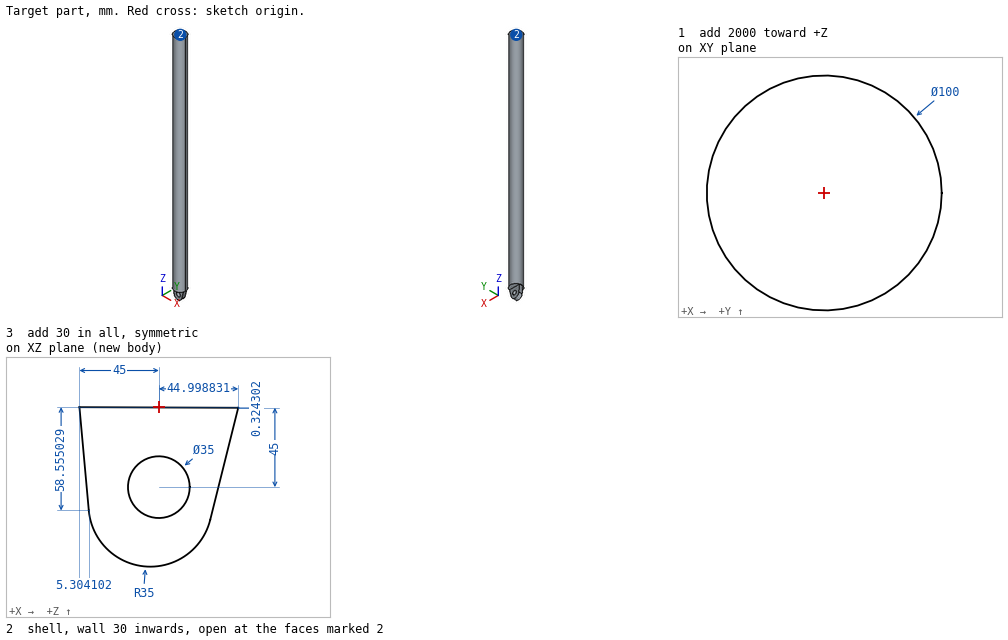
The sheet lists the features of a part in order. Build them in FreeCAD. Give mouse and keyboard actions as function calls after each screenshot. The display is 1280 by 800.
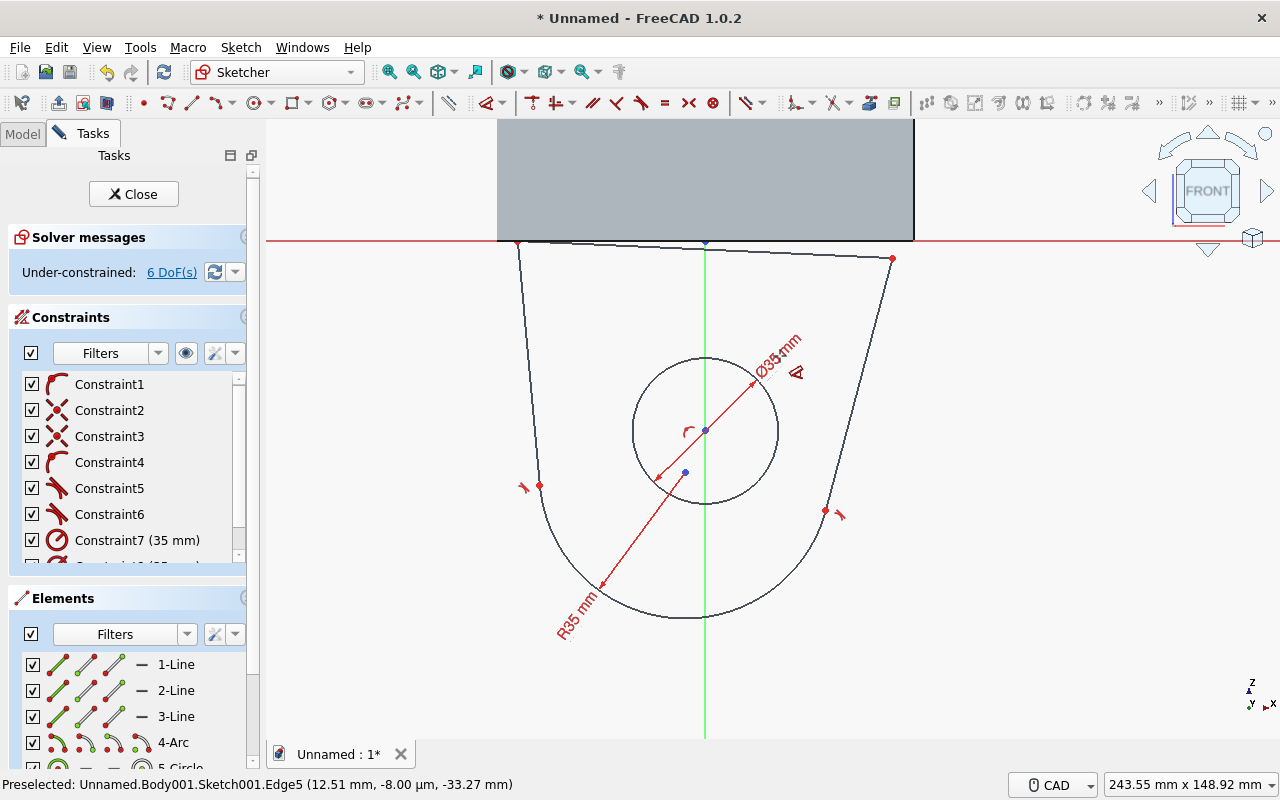
click(518, 241)
click(612, 207)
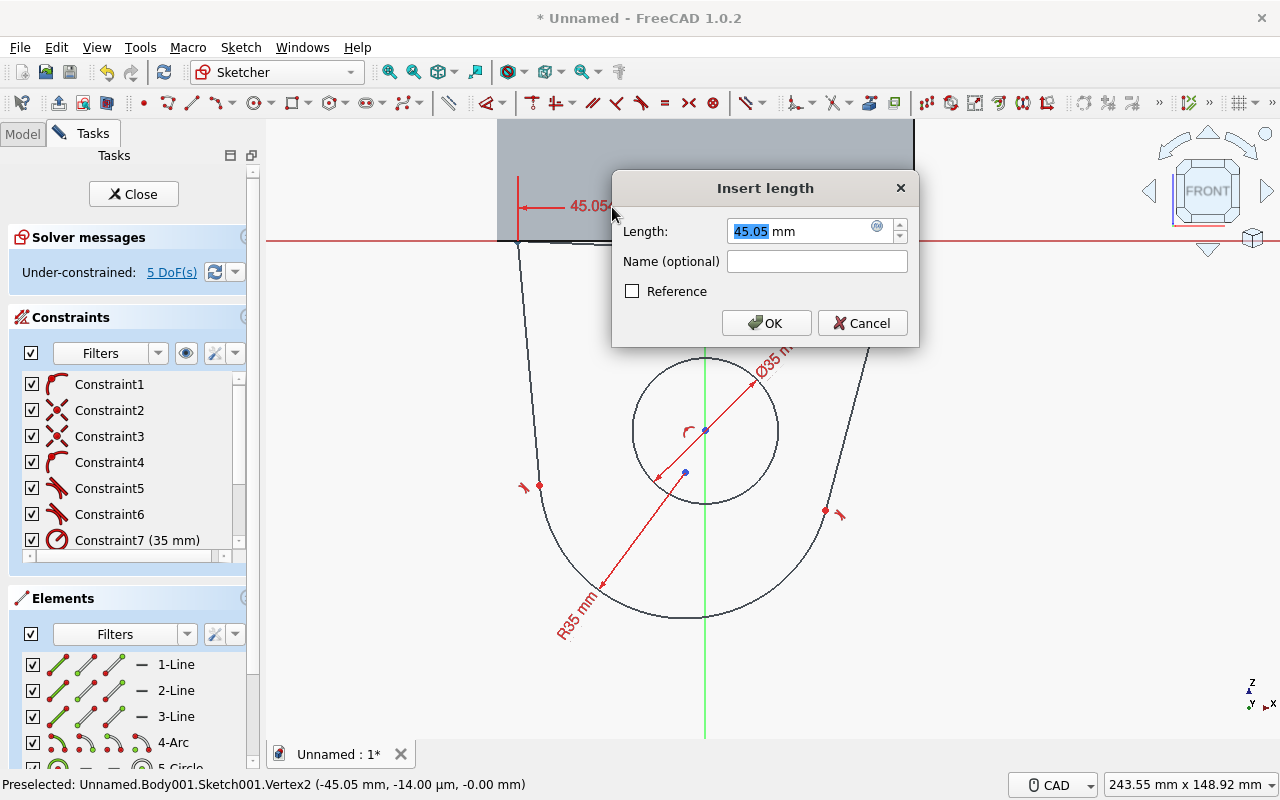
text(45)
key(Return)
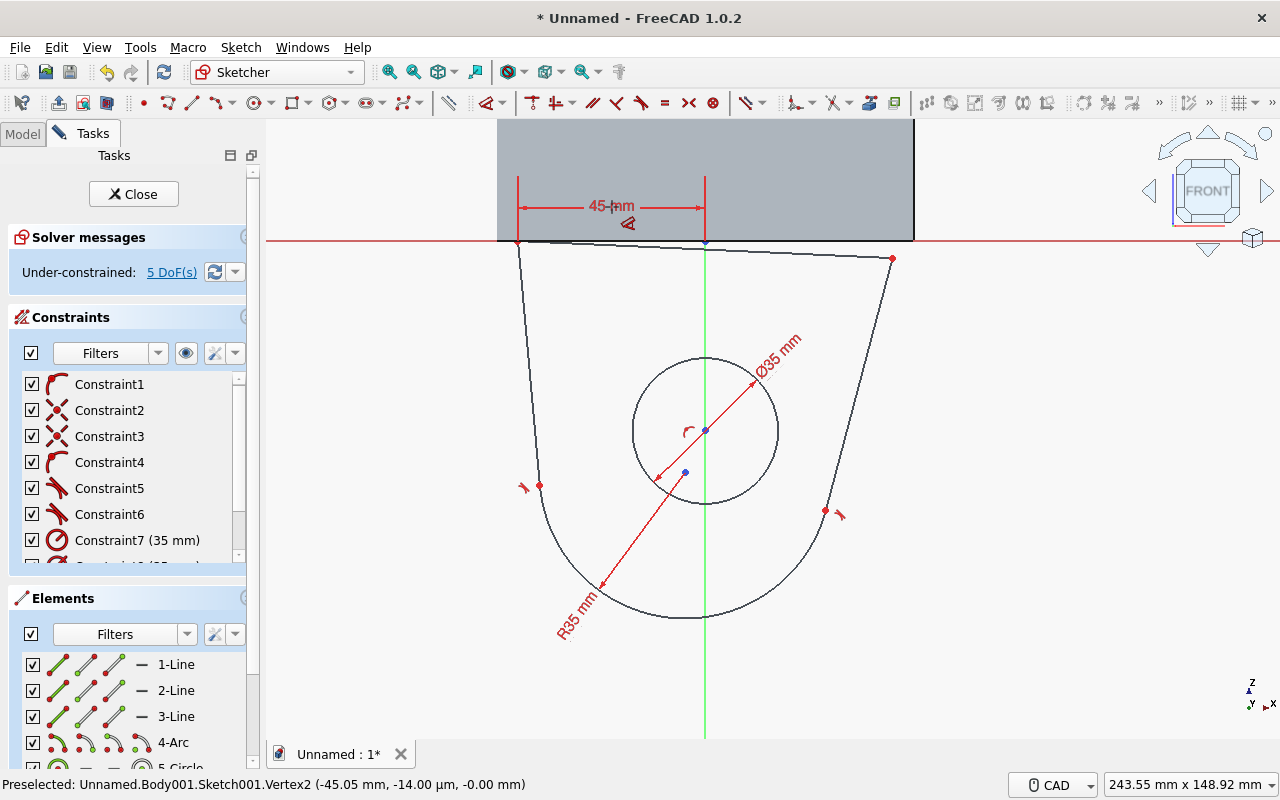
click(893, 258)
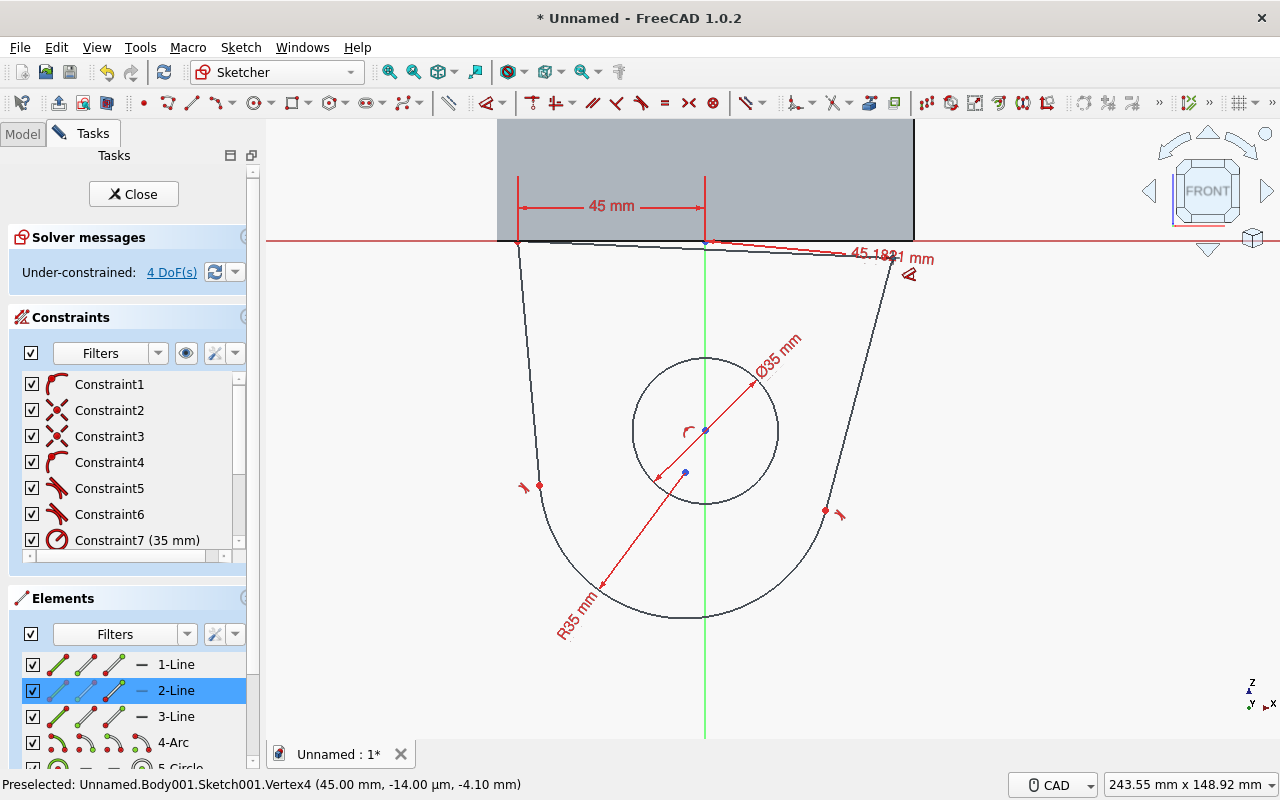
click(705, 431)
click(927, 345)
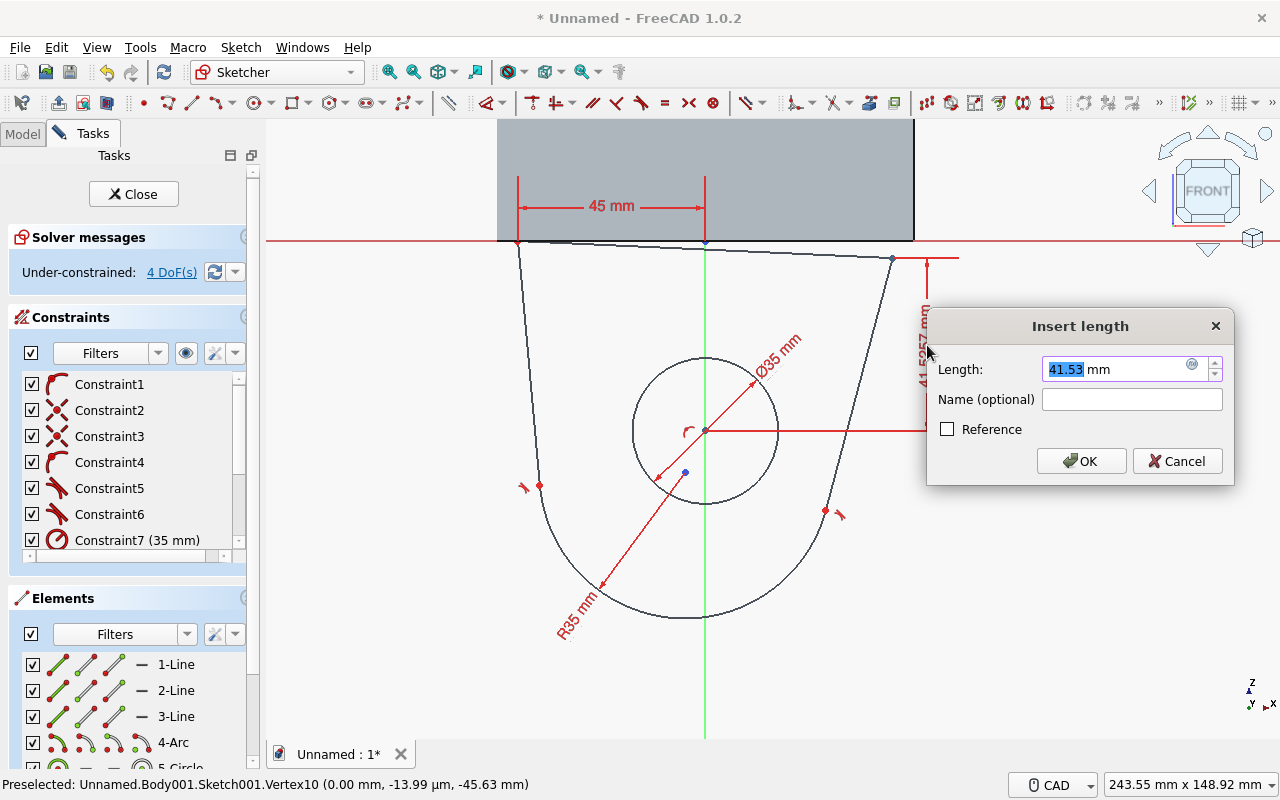
text(45)
key(Return)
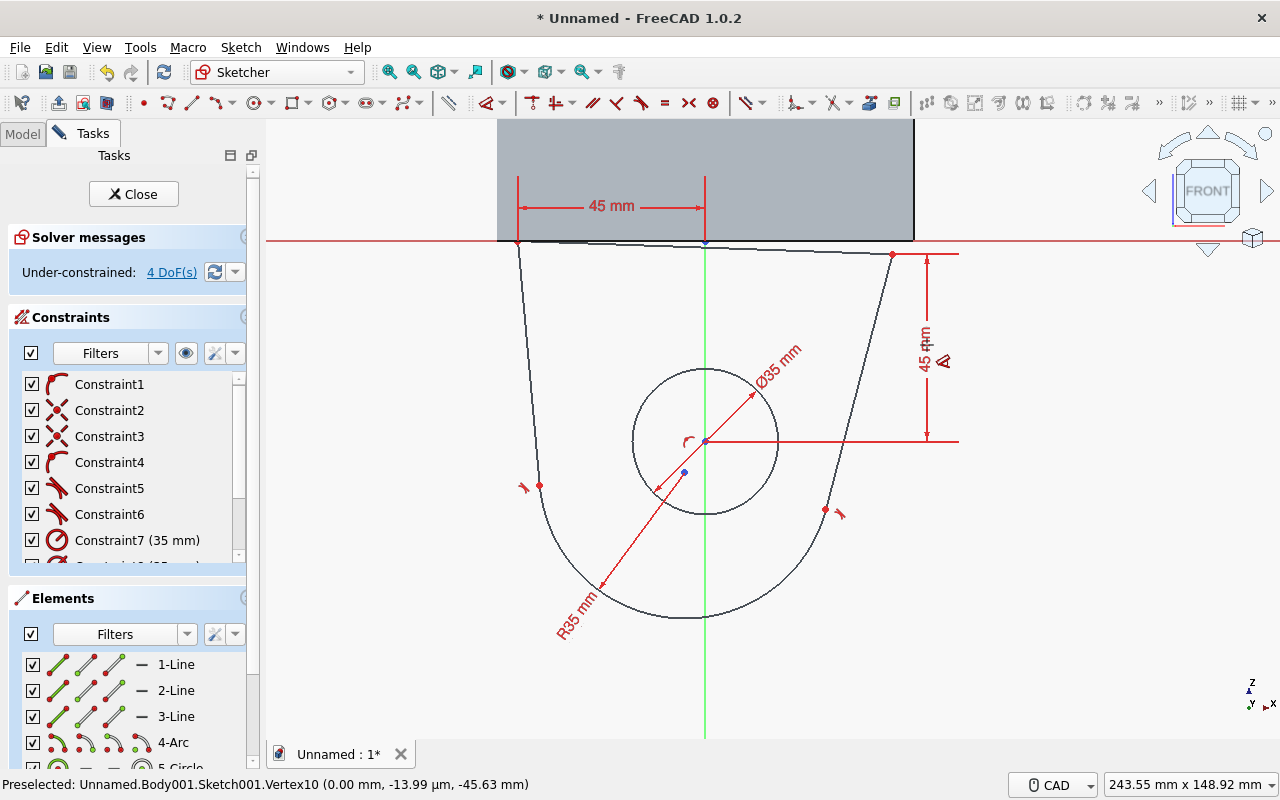
scroll(893, 254, up, 17)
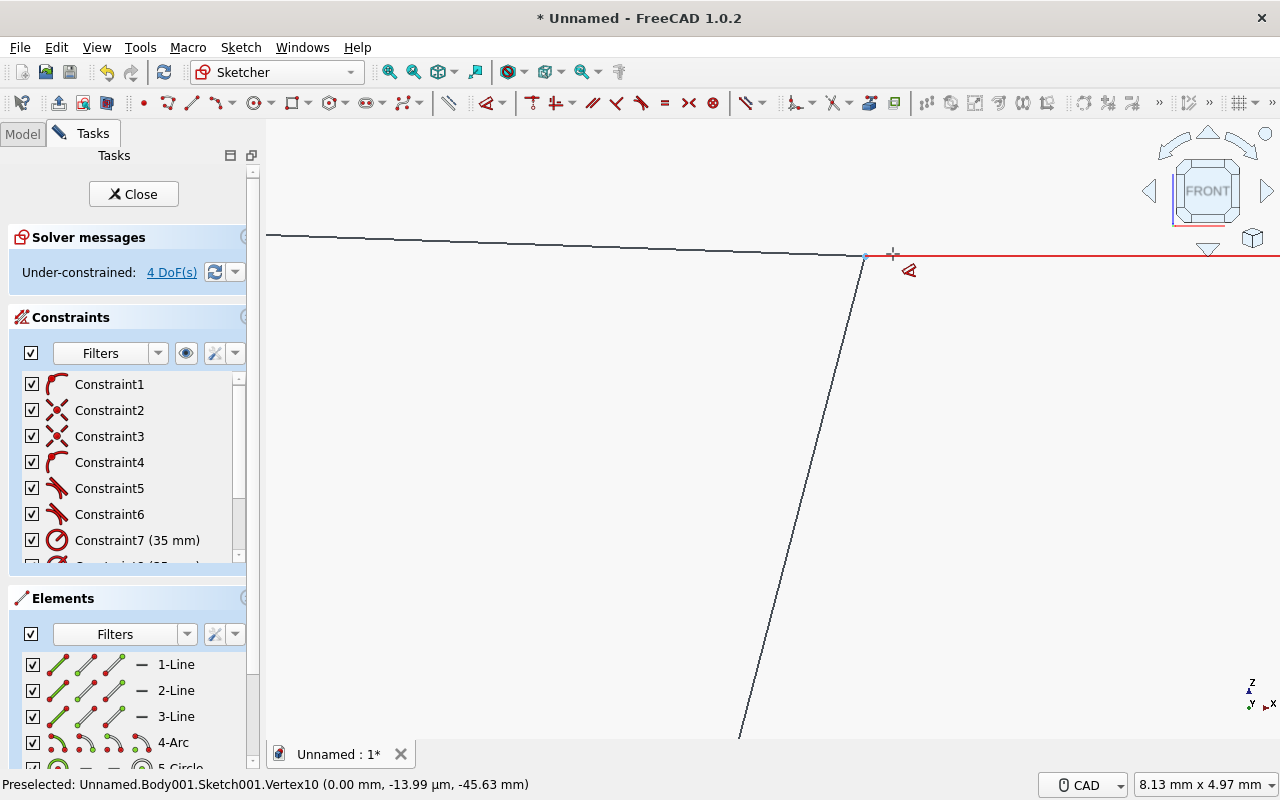
click(865, 256)
click(899, 202)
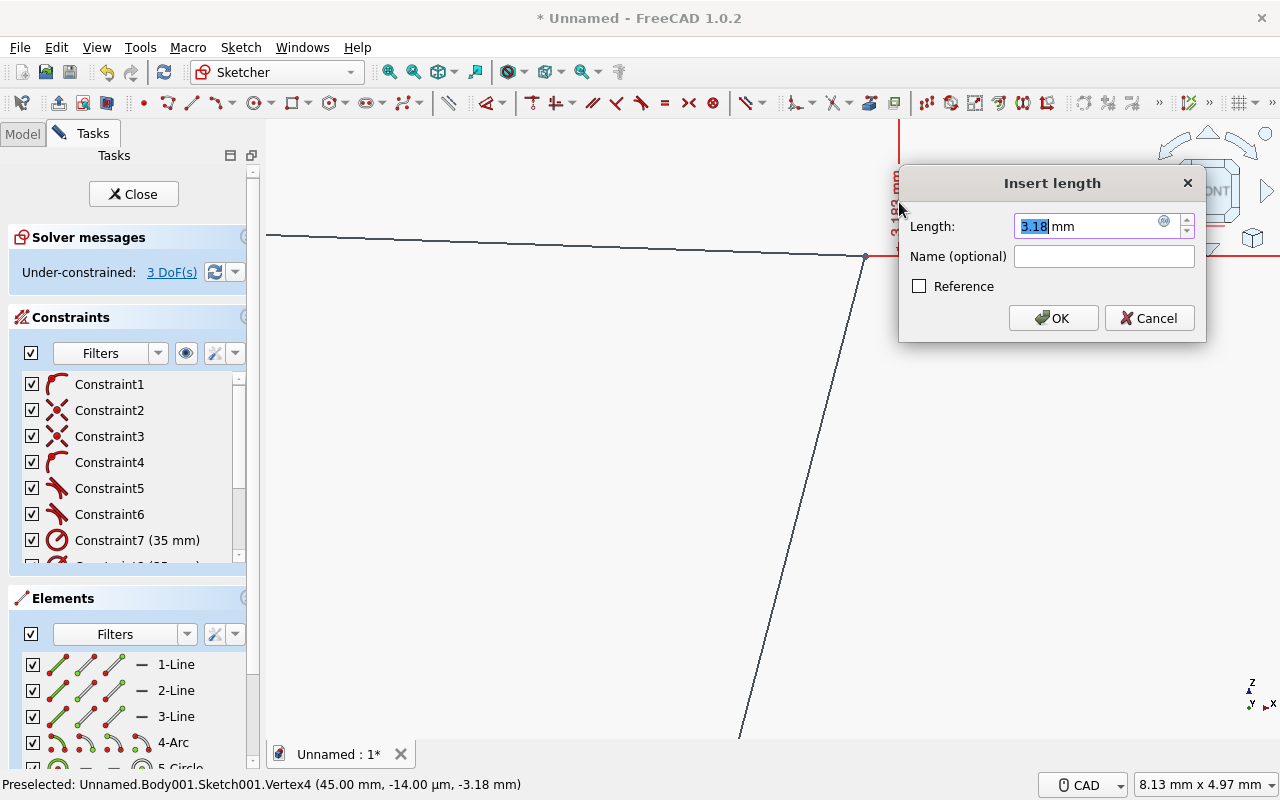
text(0.324302)
key(Return)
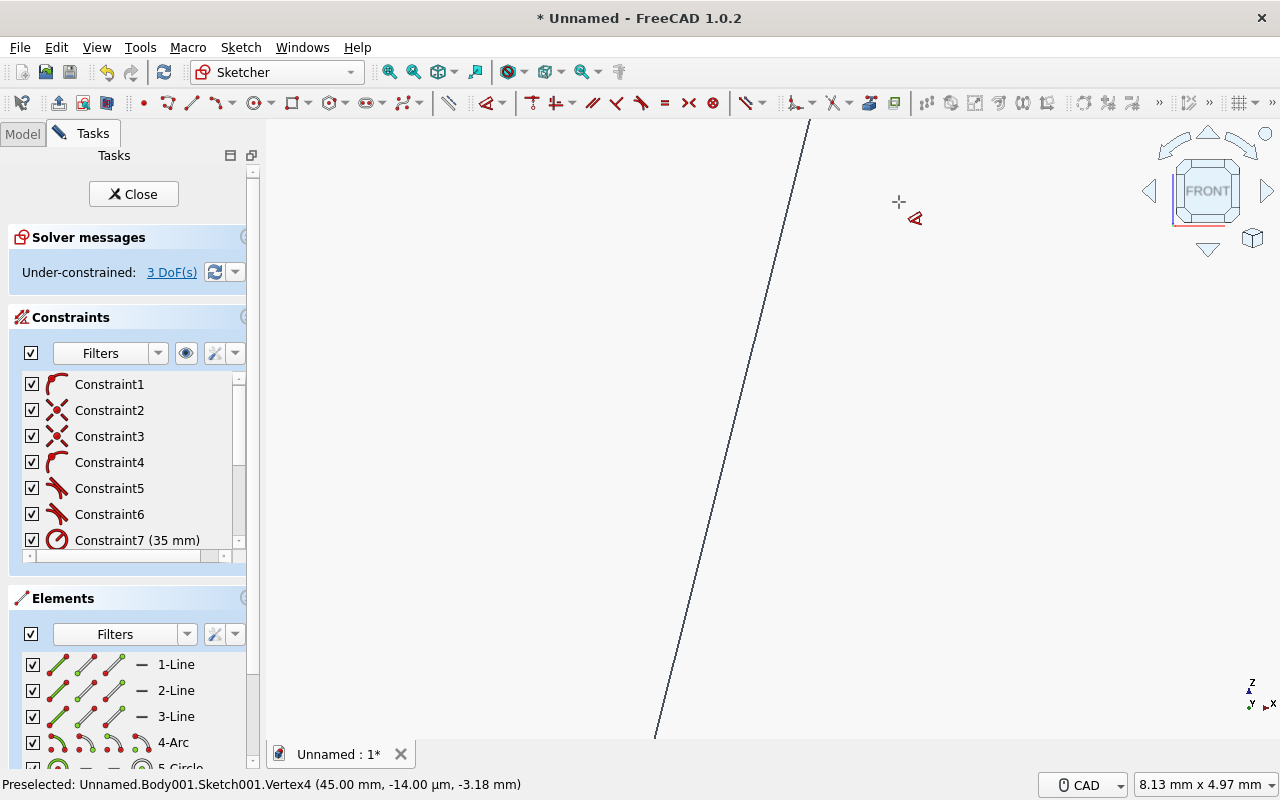
scroll(936, 214, down, 16)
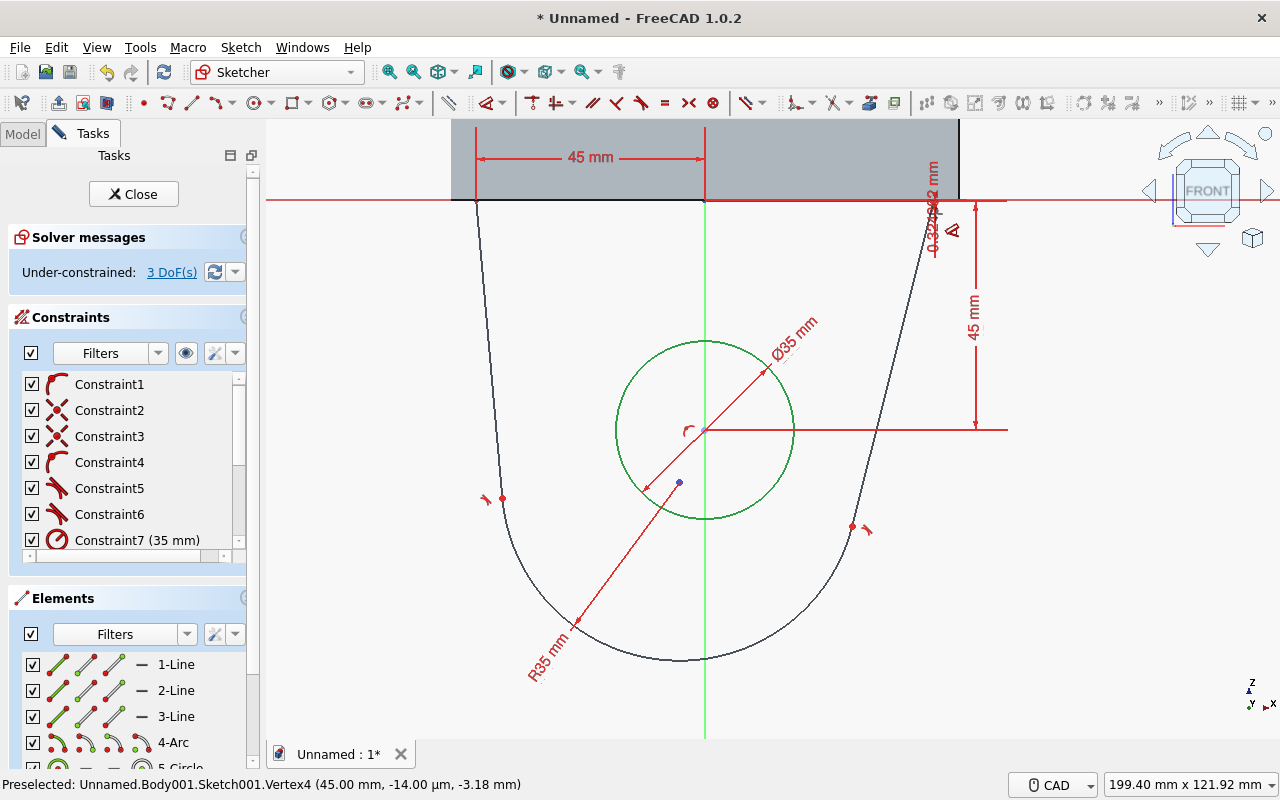
scroll(494, 409, up, 2)